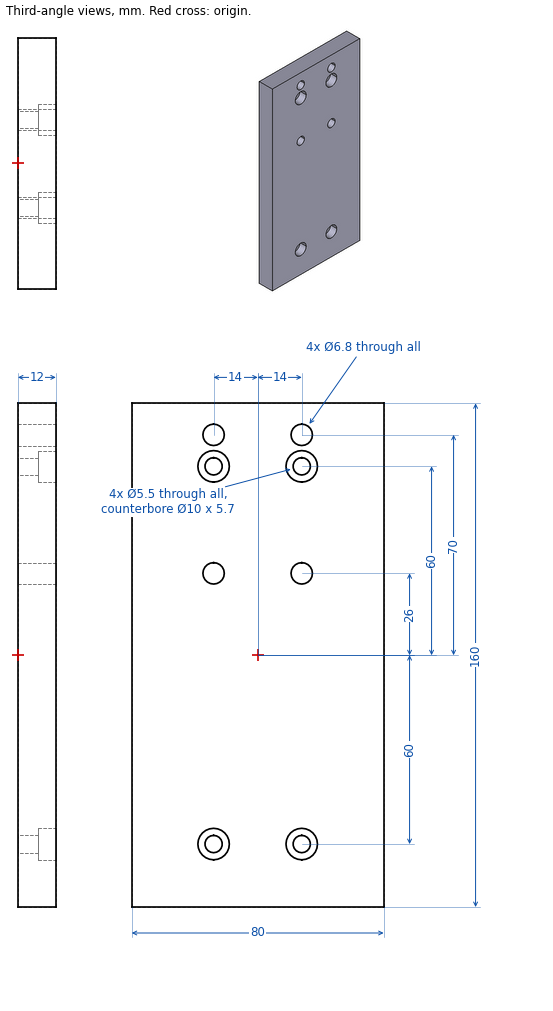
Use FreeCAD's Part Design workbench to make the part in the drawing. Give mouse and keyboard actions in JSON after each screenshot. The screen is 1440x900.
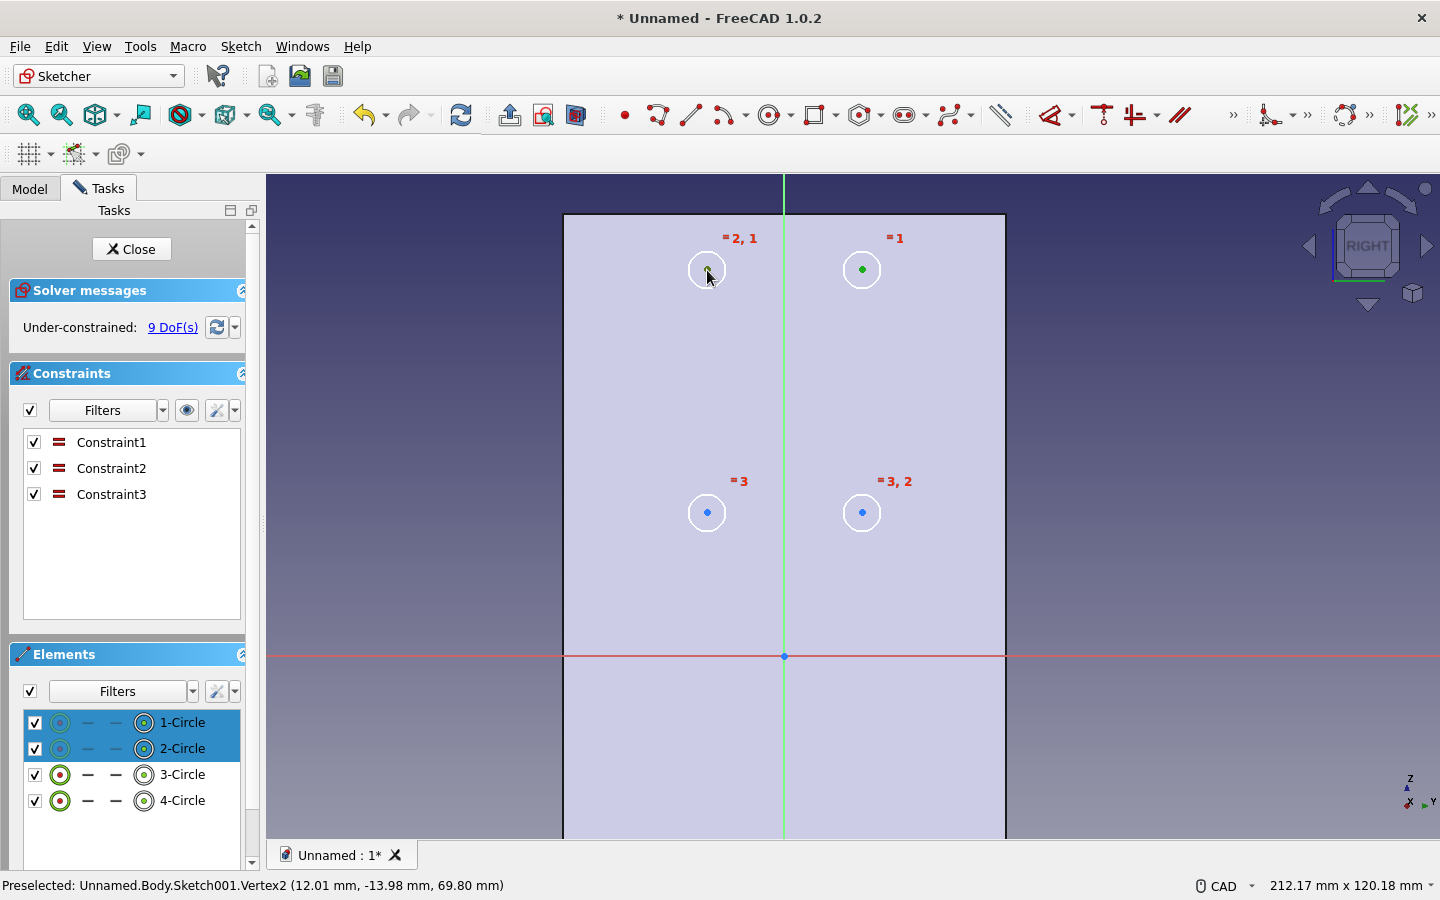
{"action": "key", "text": "h"}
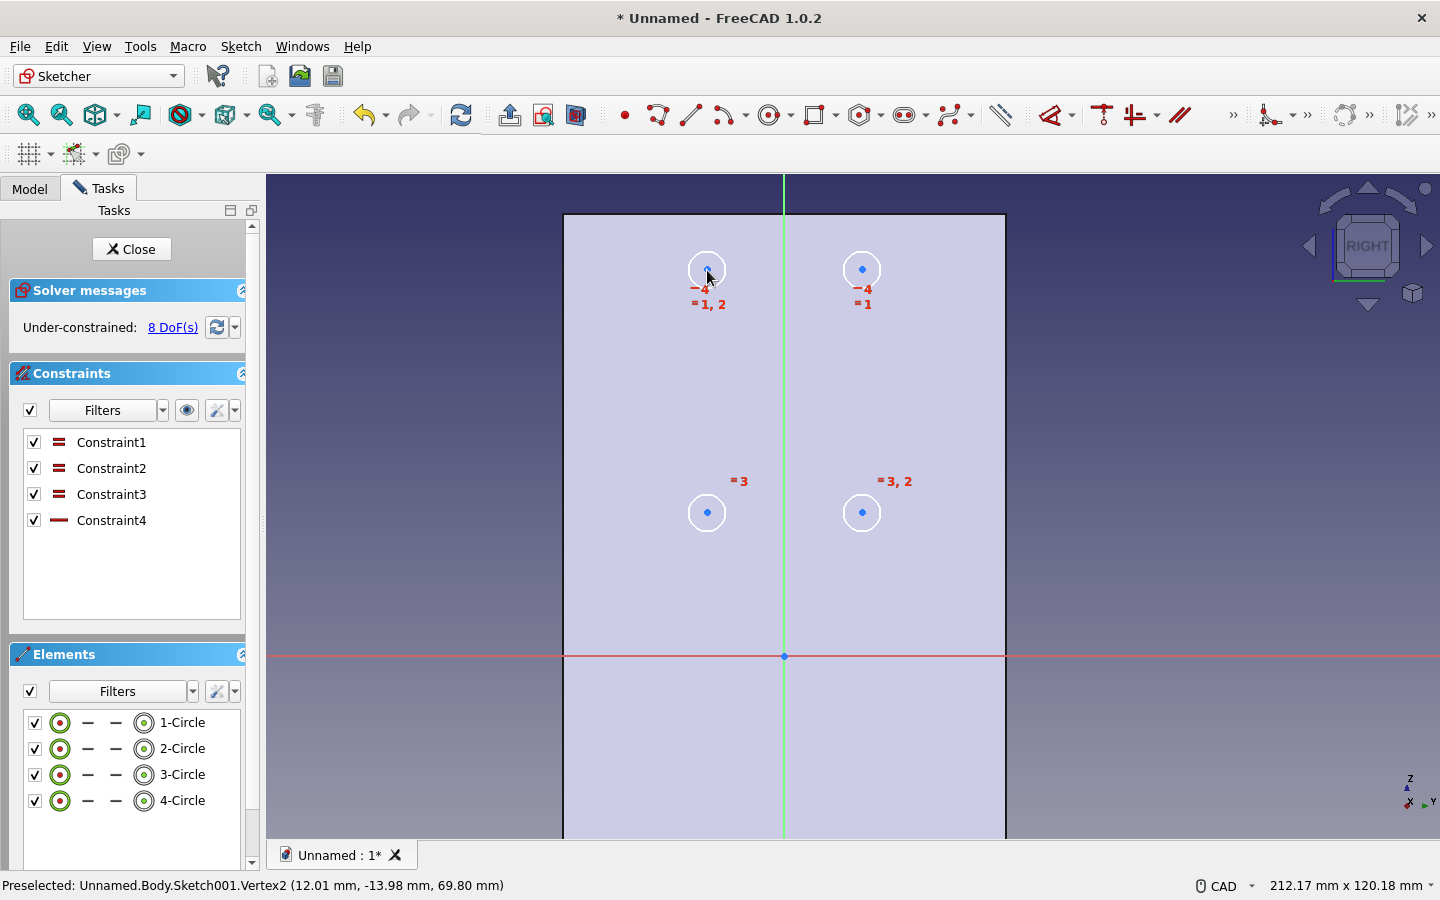
{"action": "left_click", "coordinate": [862, 270]}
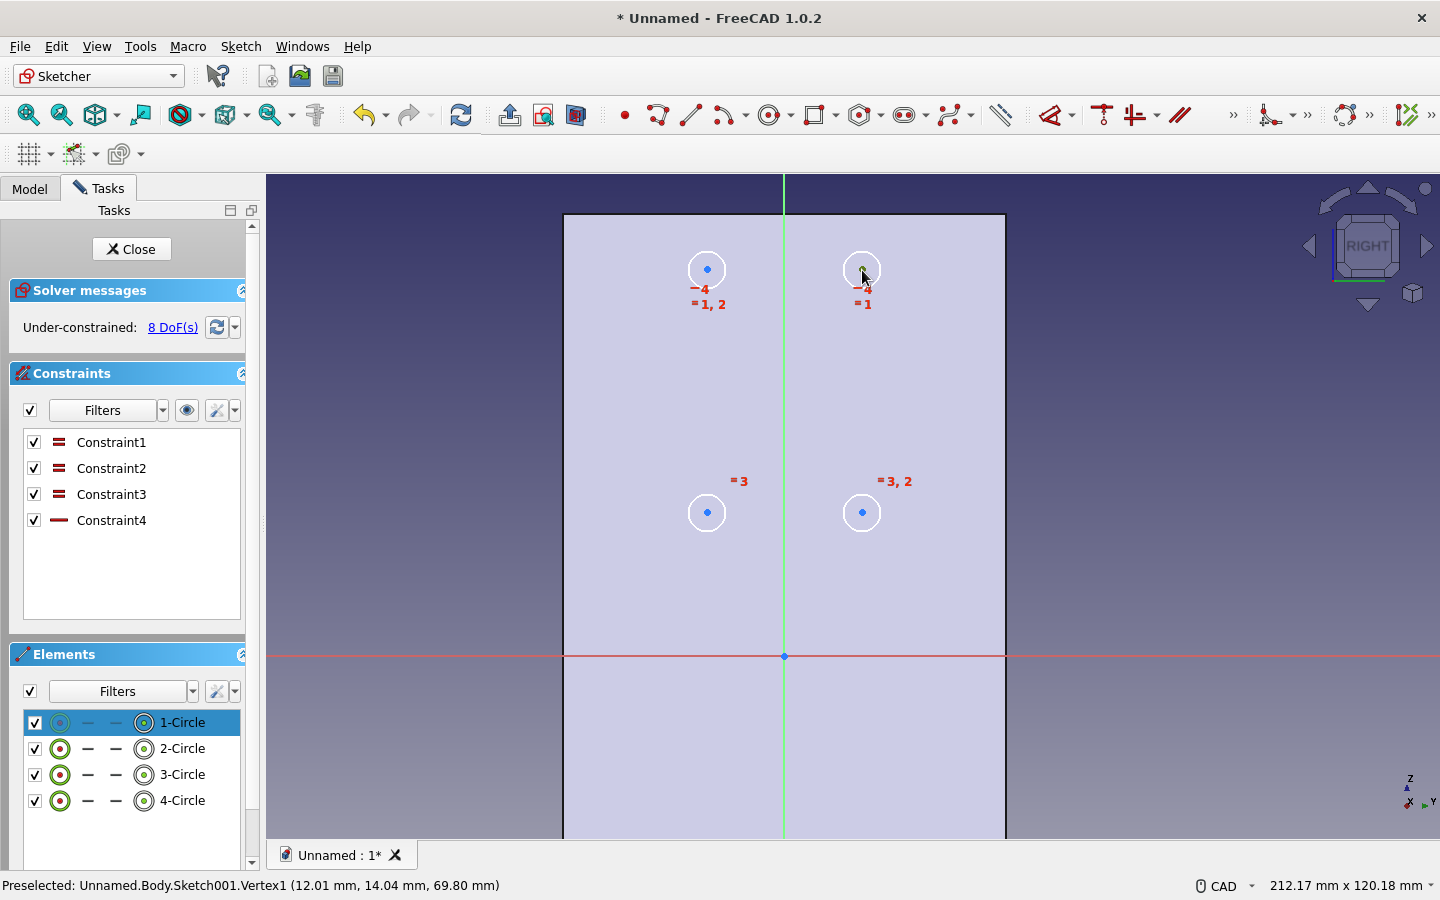
{"action": "left_click", "coordinate": [862, 513]}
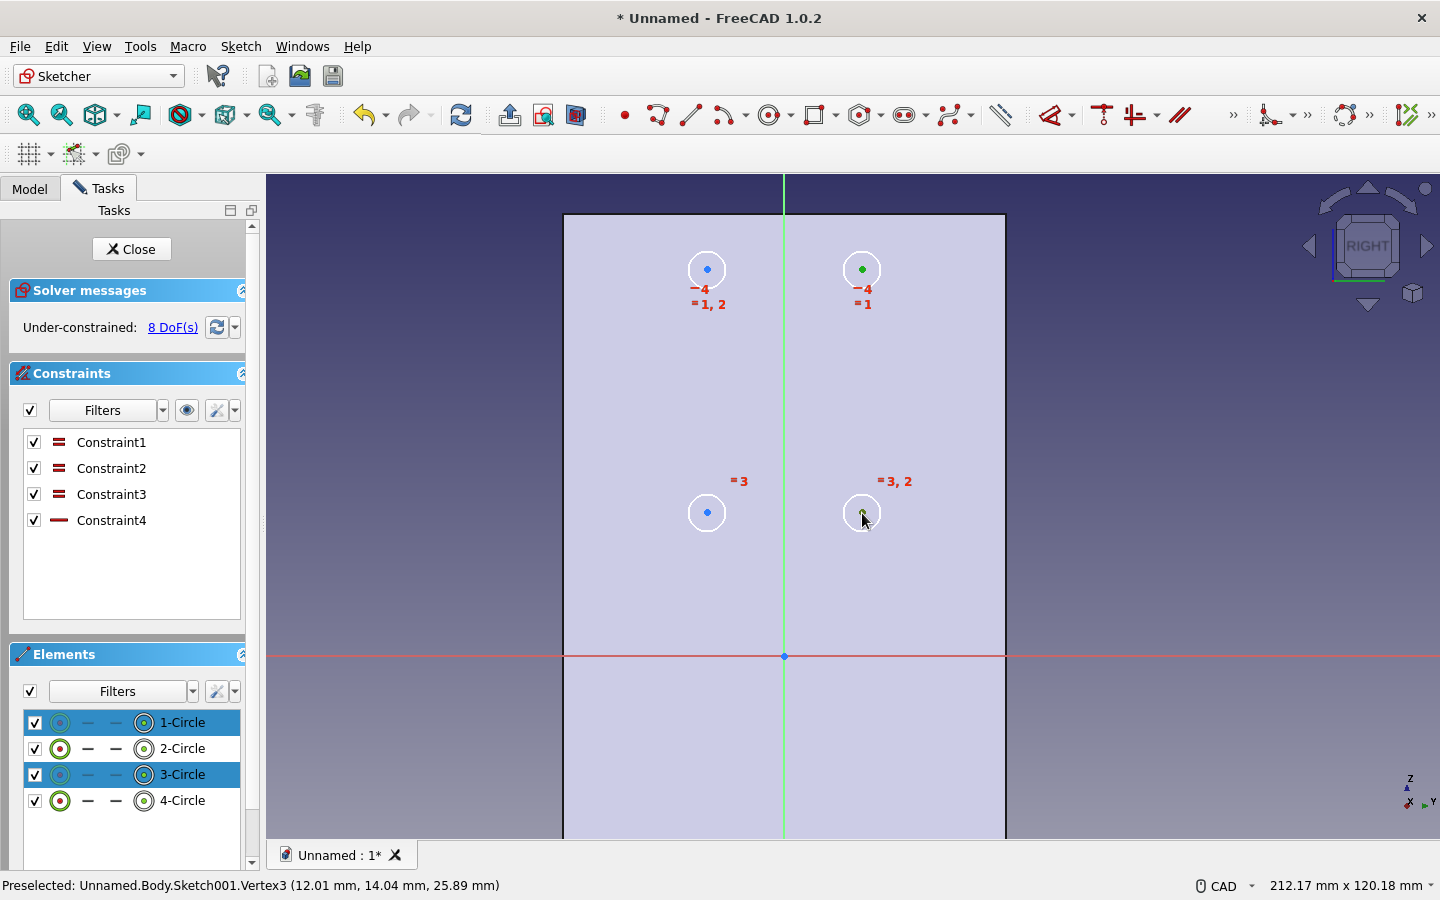
{"action": "left_click", "coordinate": [1156, 116]}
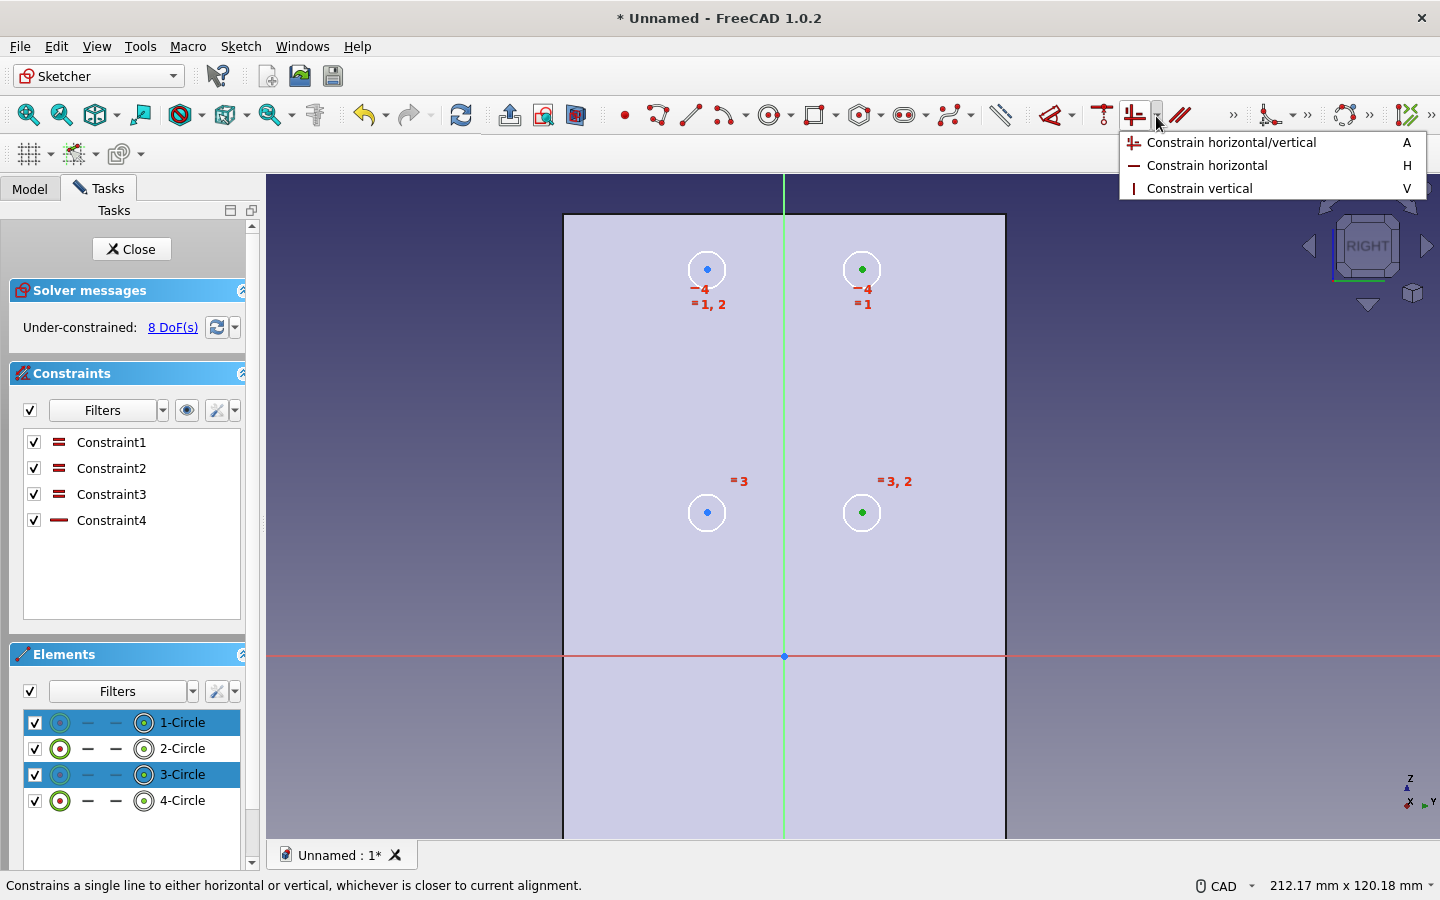
{"action": "left_click", "coordinate": [1273, 188]}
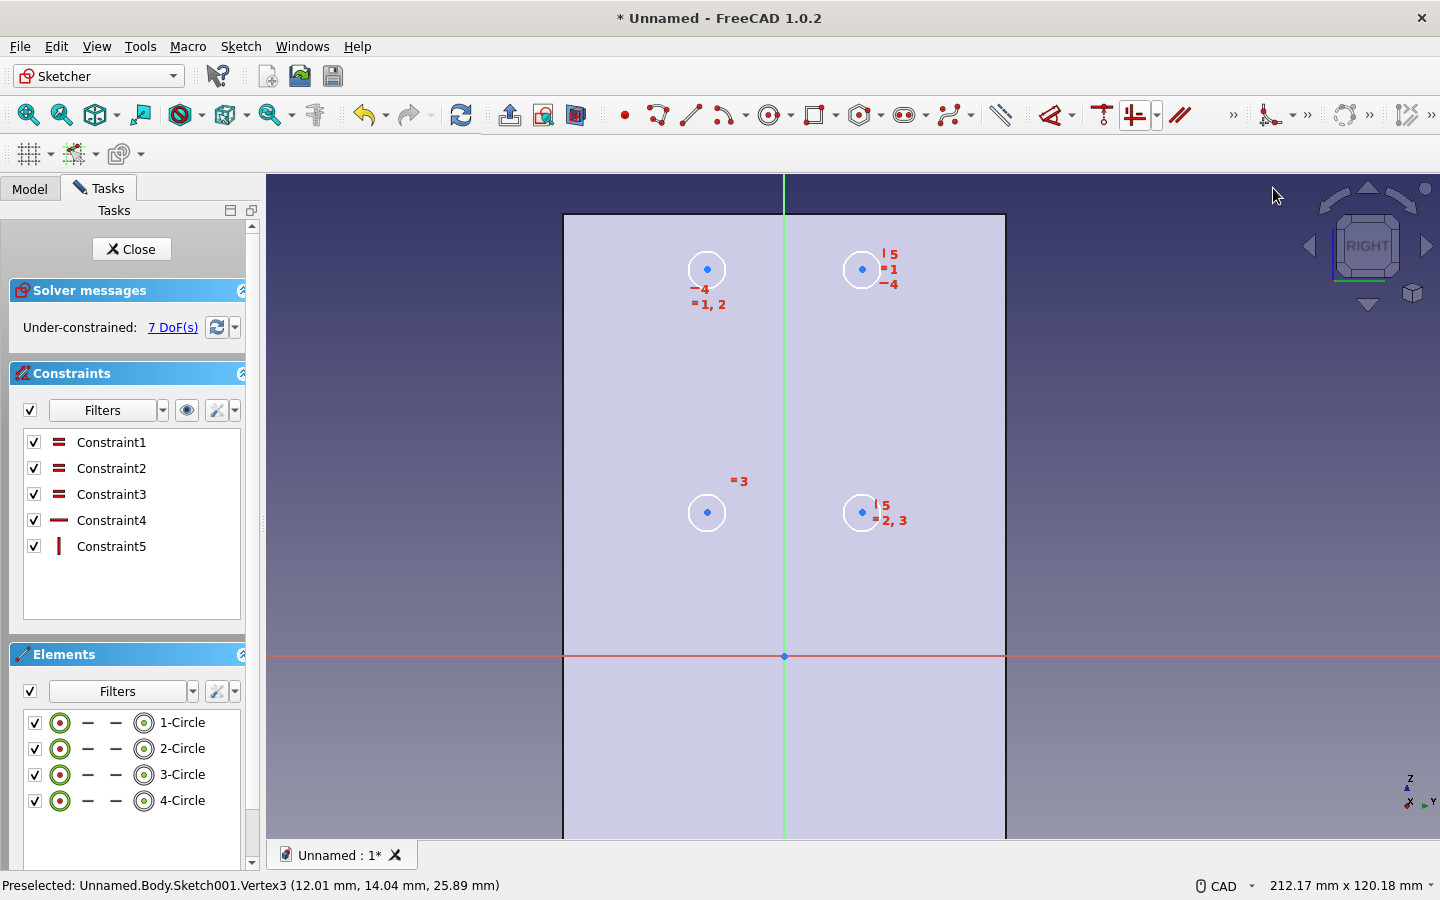
{"action": "left_click", "coordinate": [707, 270]}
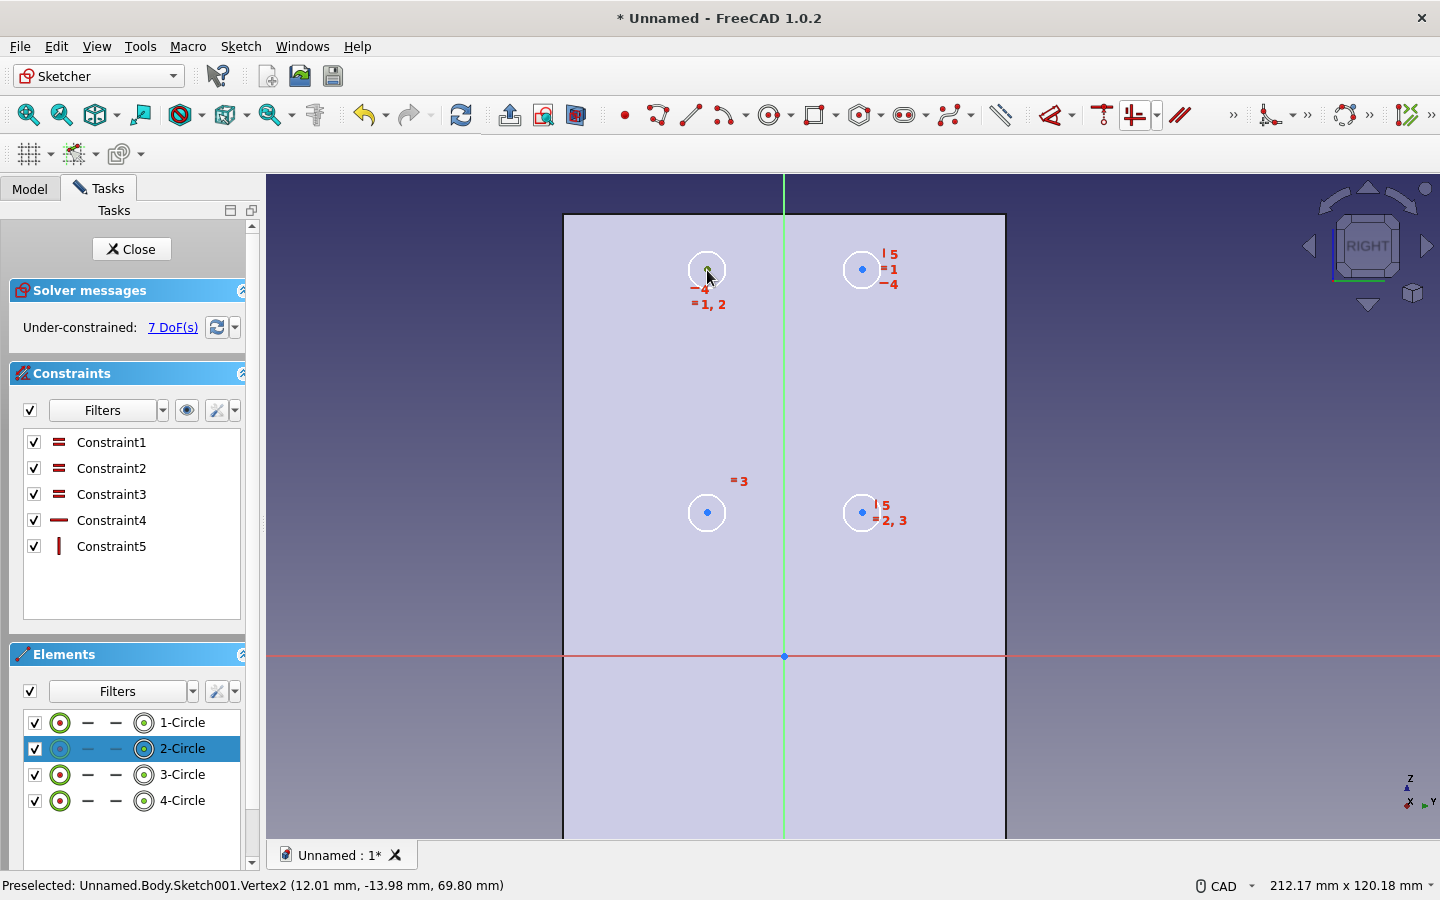
{"action": "left_click", "coordinate": [707, 513]}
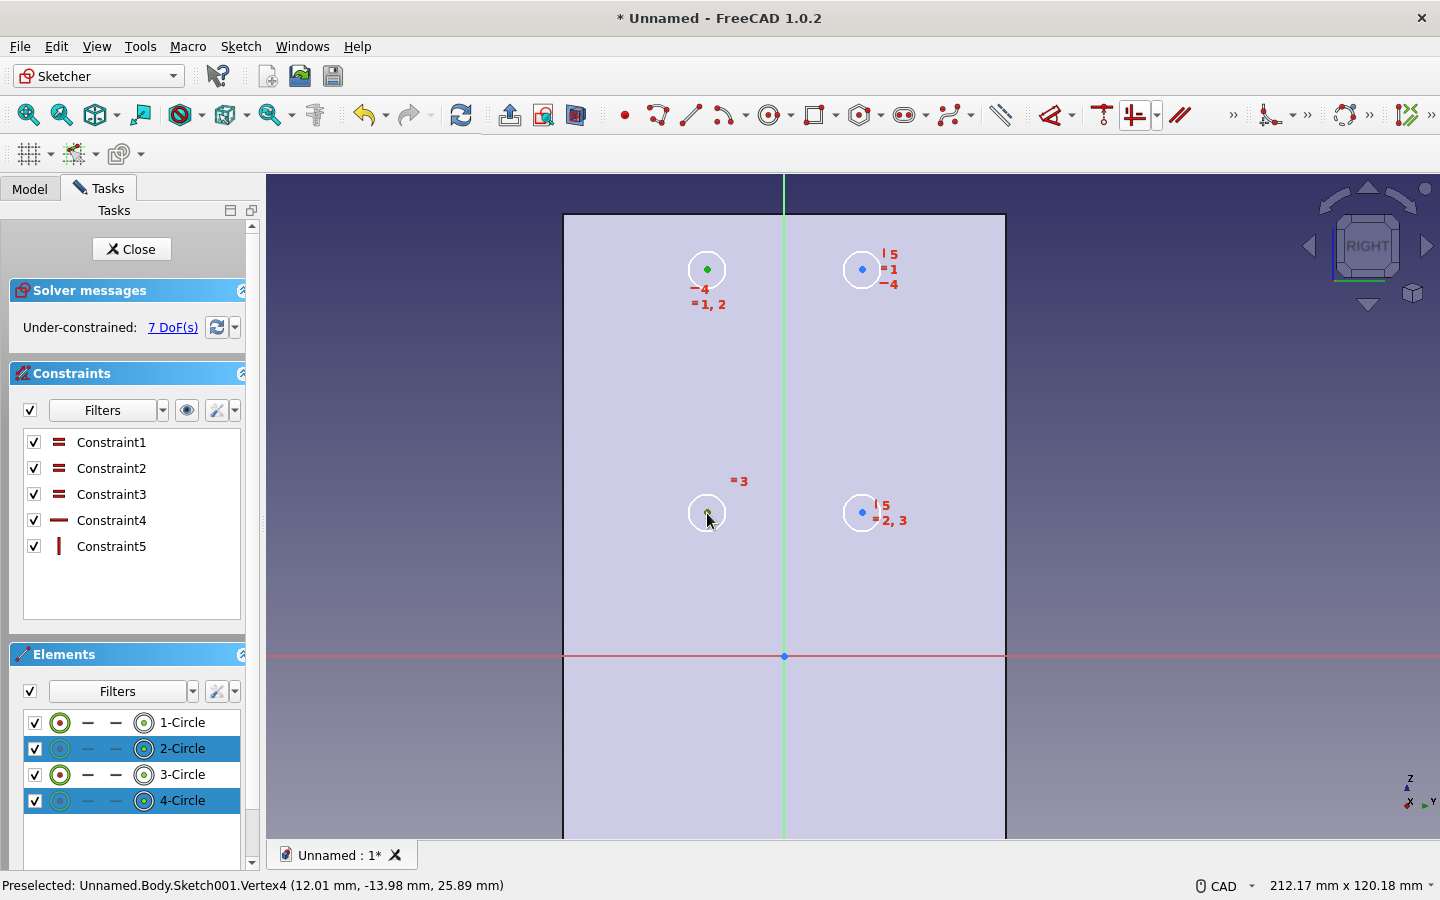
{"action": "key", "text": "v"}